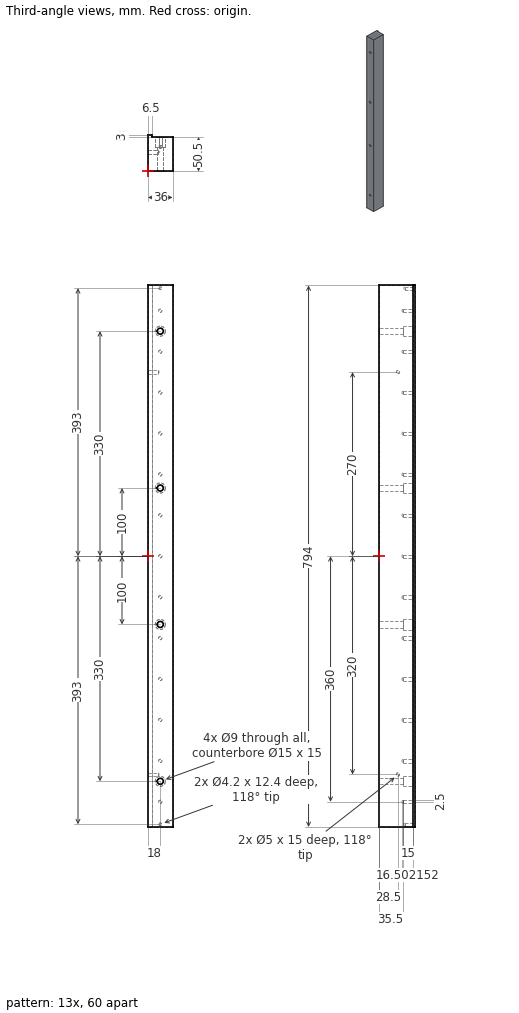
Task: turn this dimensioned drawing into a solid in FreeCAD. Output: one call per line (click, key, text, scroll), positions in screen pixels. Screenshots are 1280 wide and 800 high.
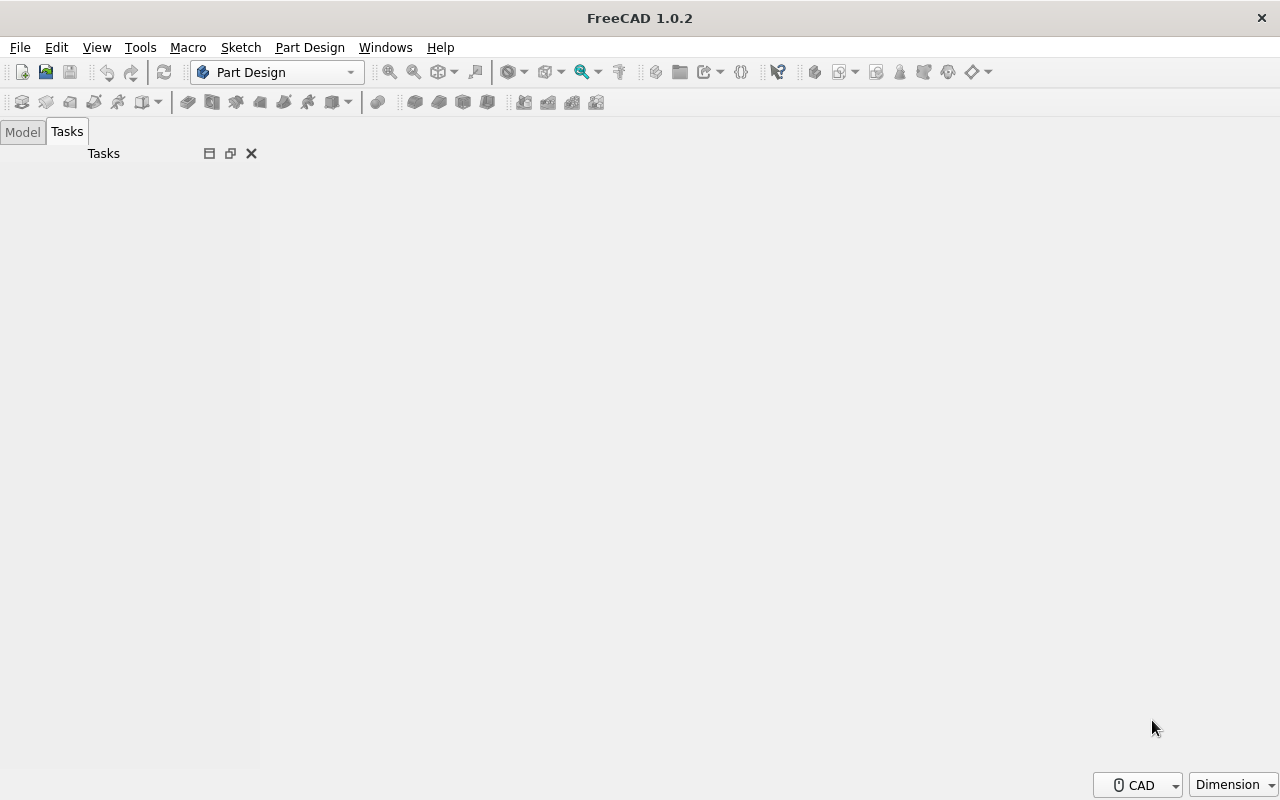
click(22, 72)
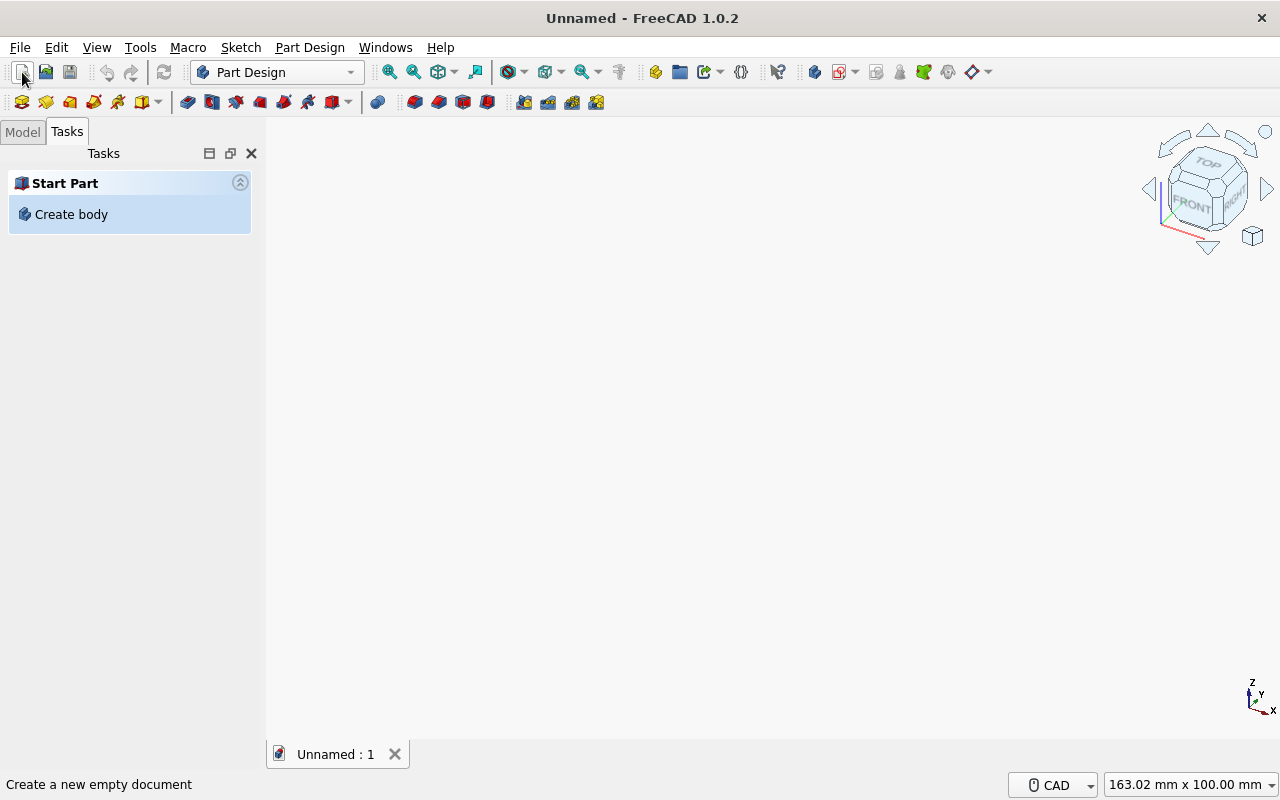
click(840, 72)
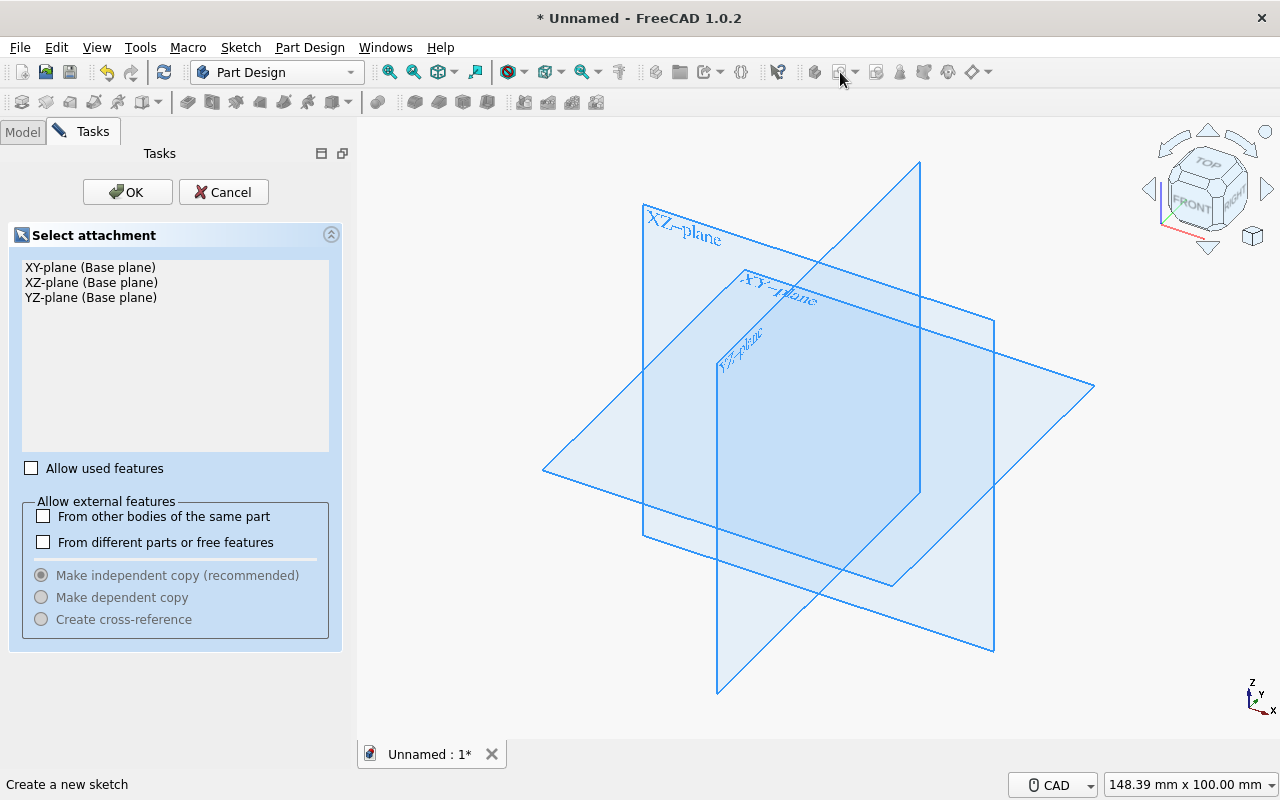
click(82, 268)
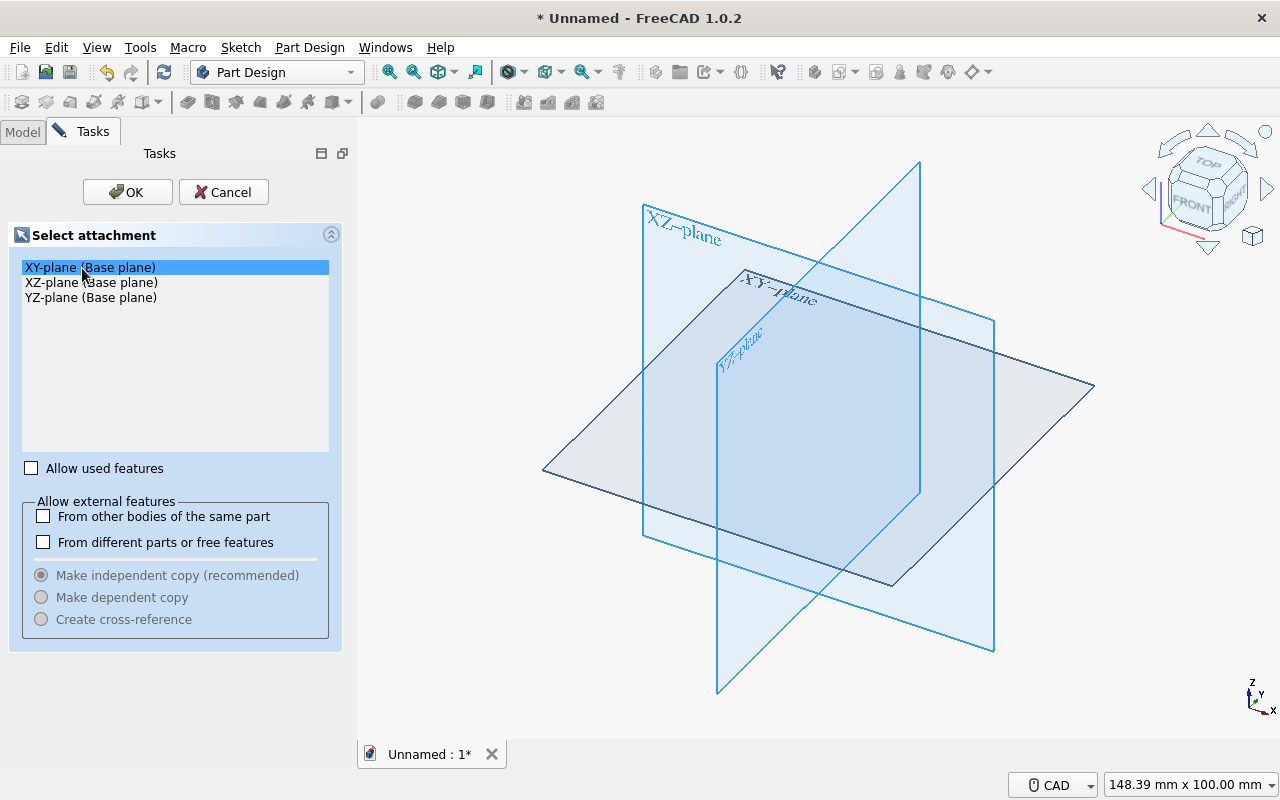
click(128, 192)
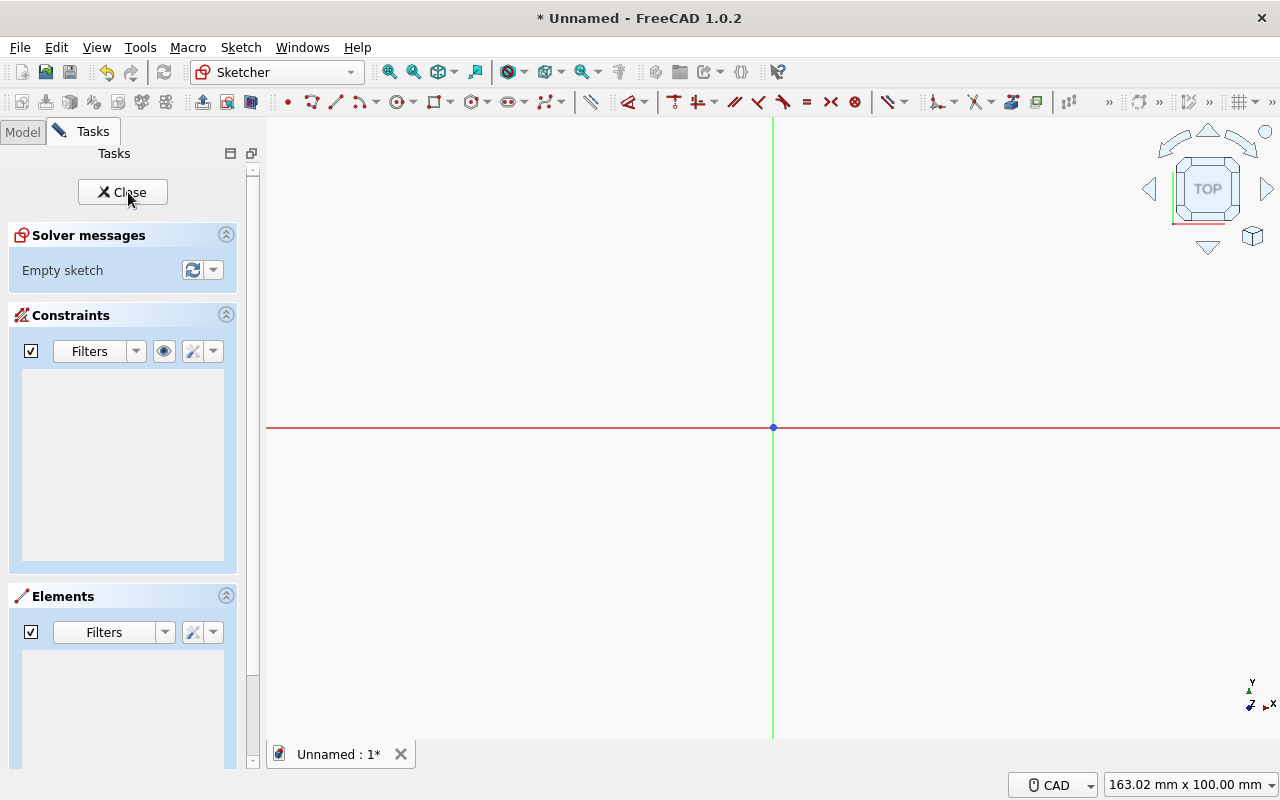
scroll(294, 711, down, 1)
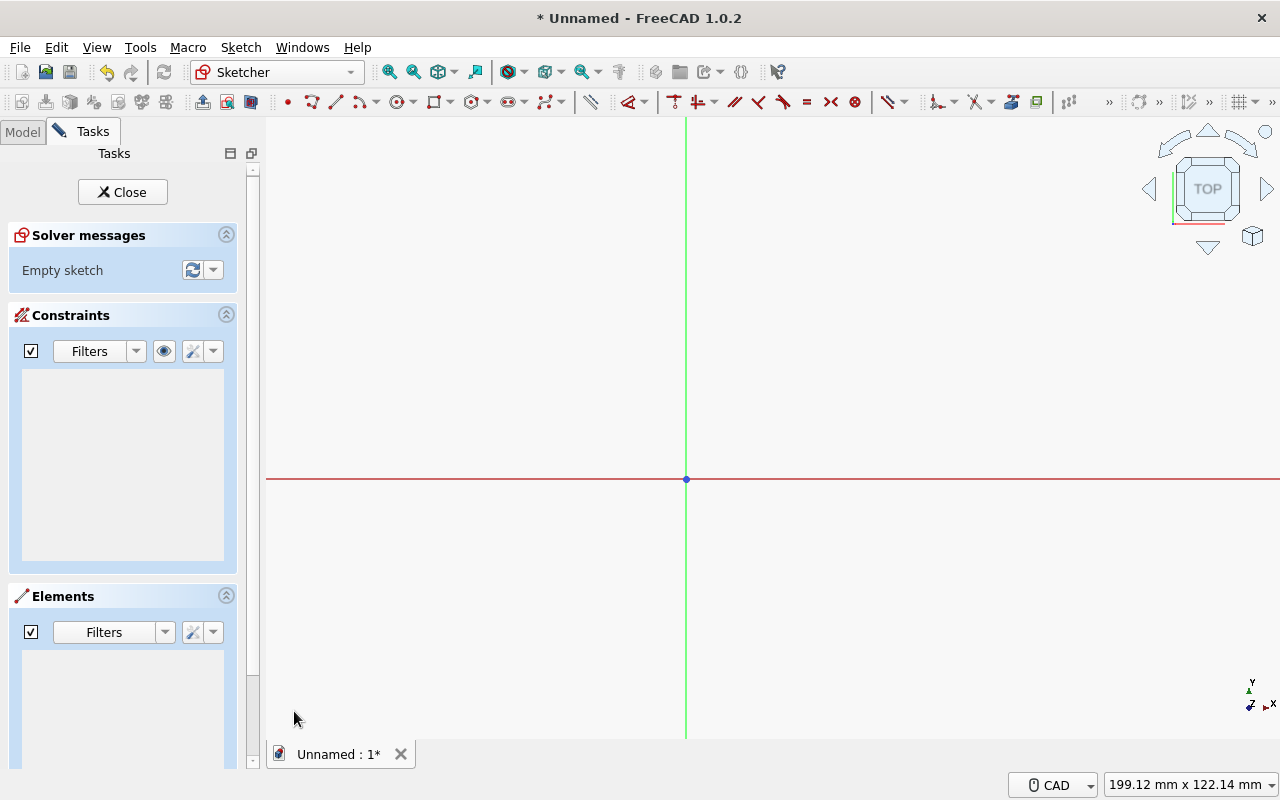
scroll(927, 171, up, 2)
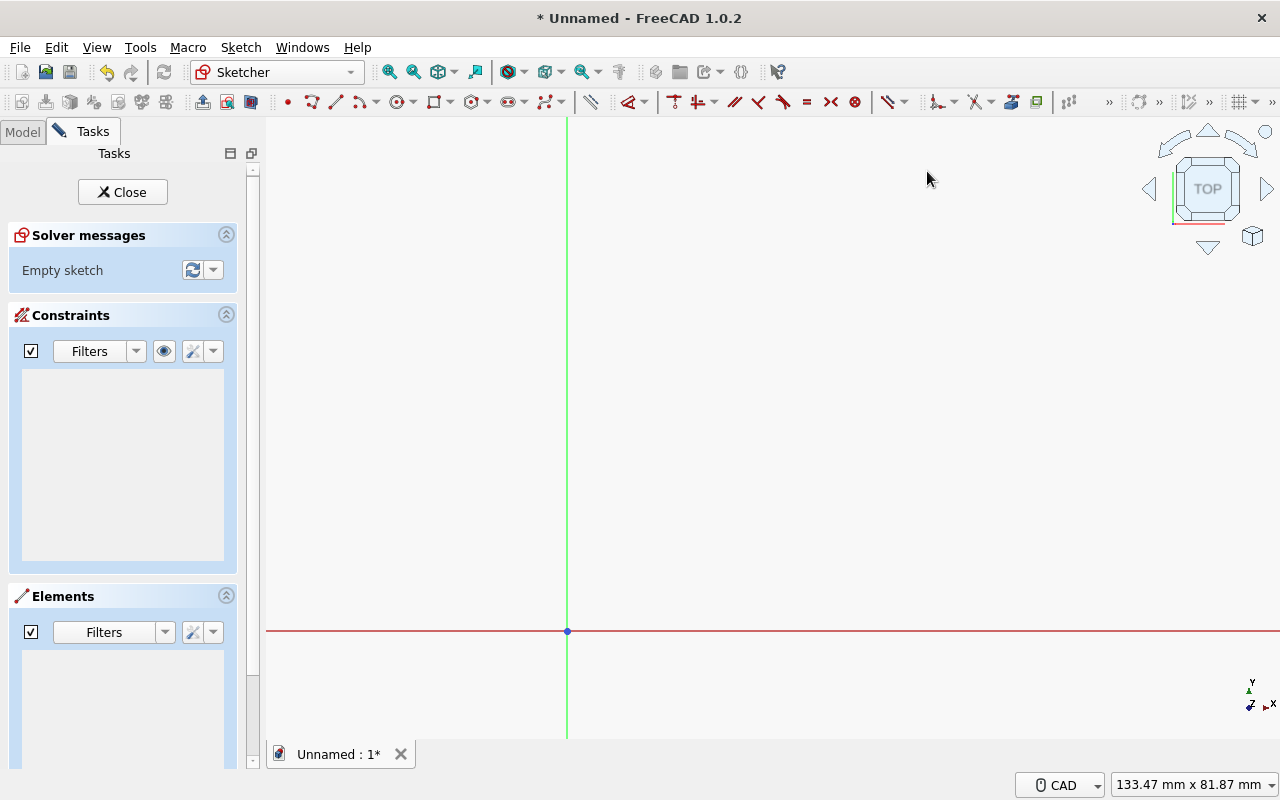
click(312, 102)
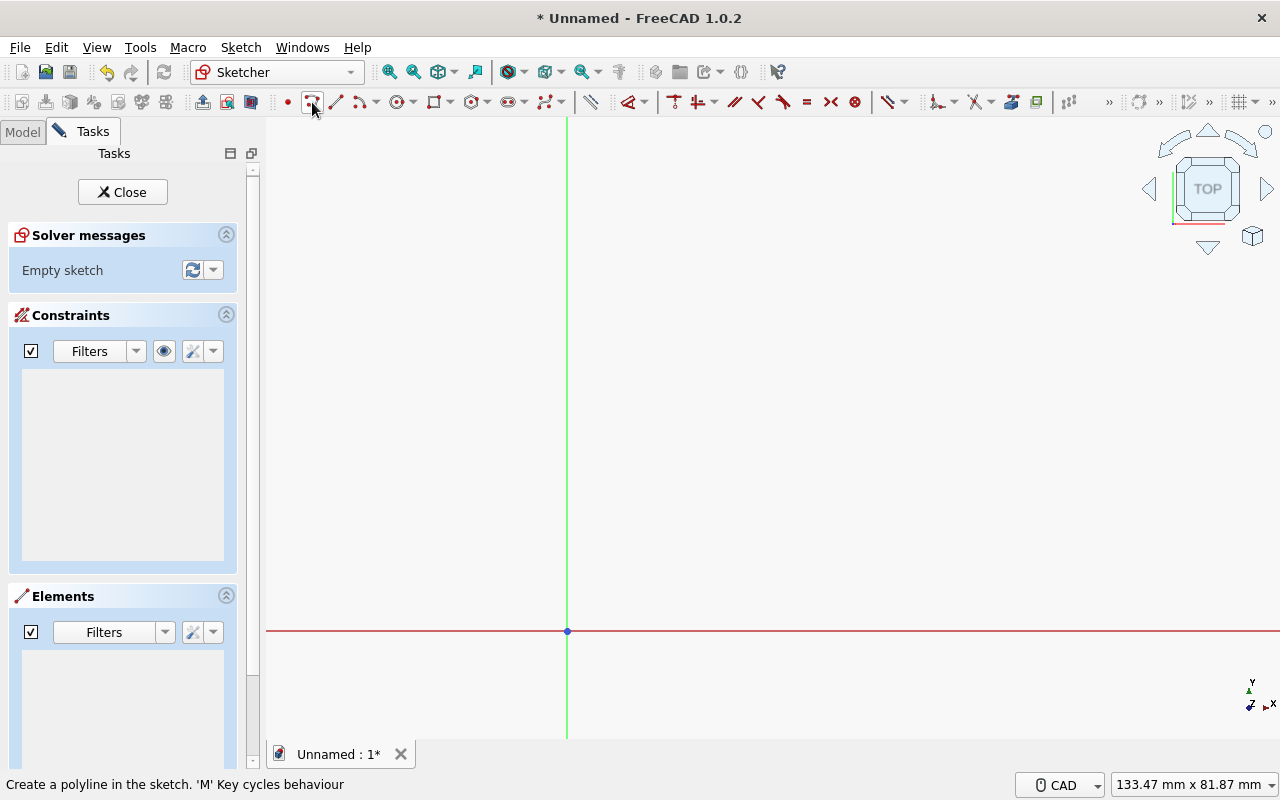
click(567, 631)
click(841, 622)
click(841, 247)
click(617, 247)
click(617, 225)
click(576, 225)
click(567, 631)
key(Escape)
key(Escape)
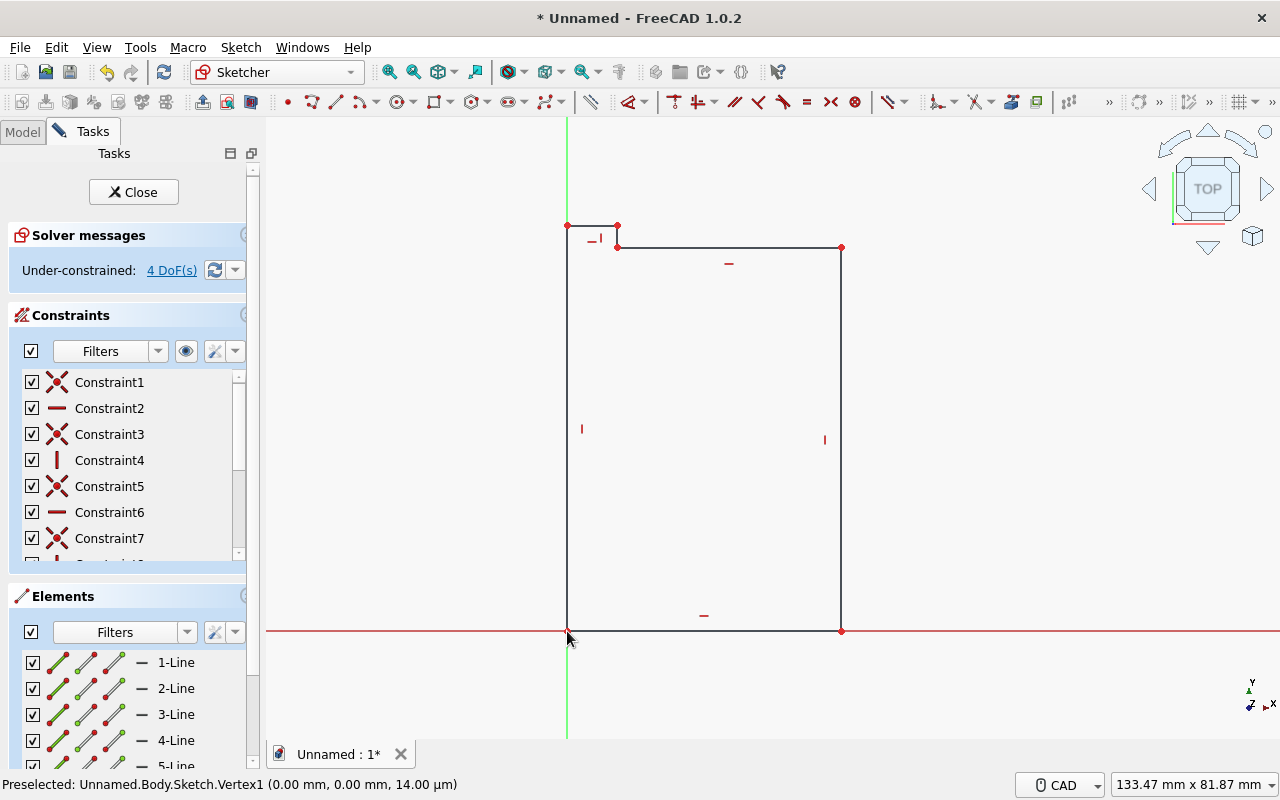
scroll(617, 237, up, 3)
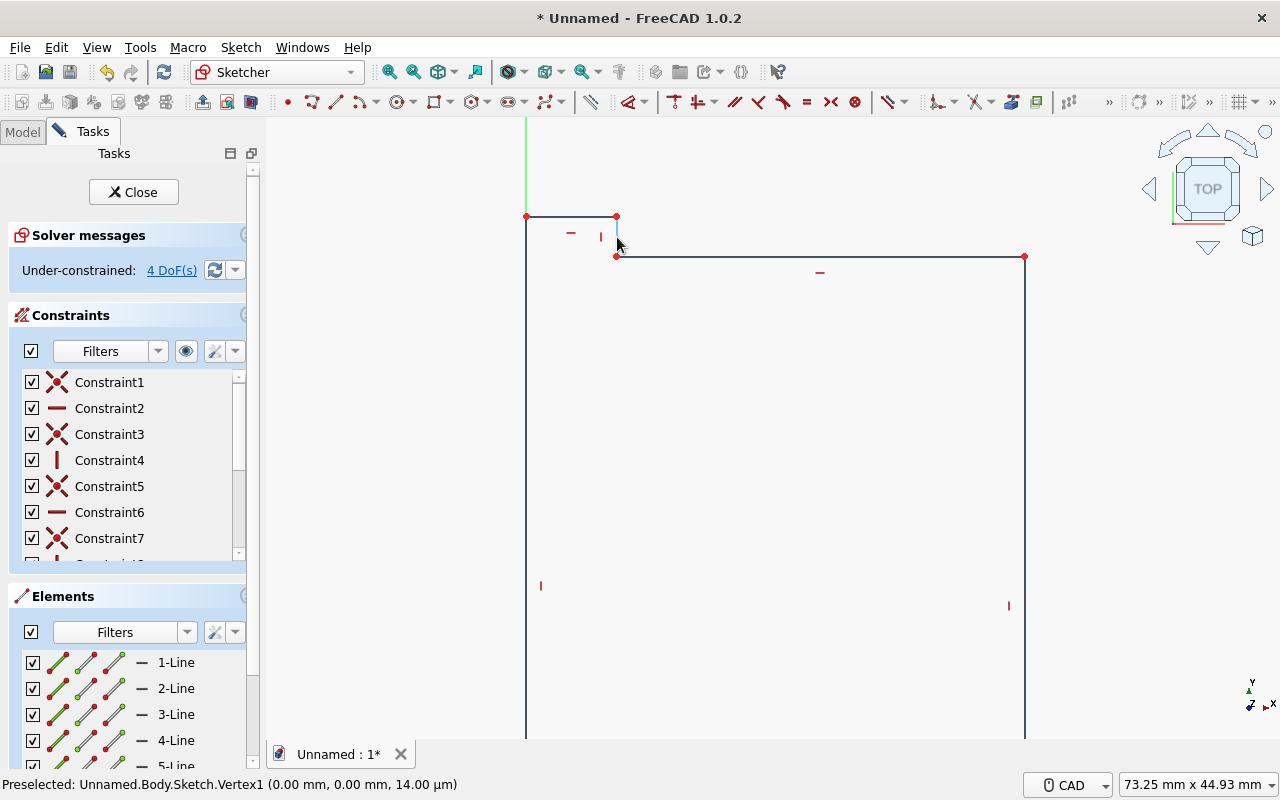
click(617, 237)